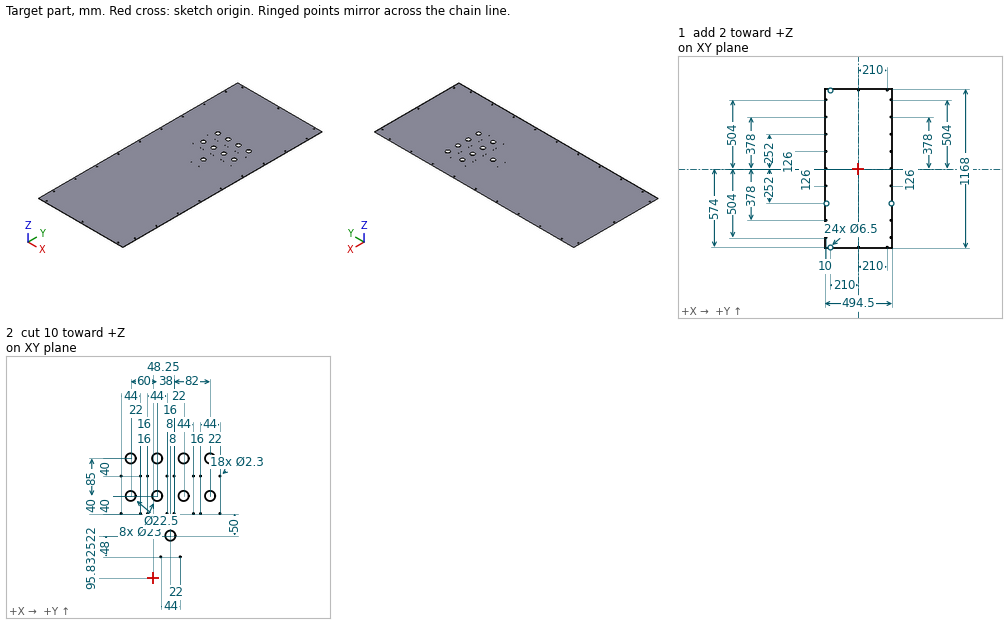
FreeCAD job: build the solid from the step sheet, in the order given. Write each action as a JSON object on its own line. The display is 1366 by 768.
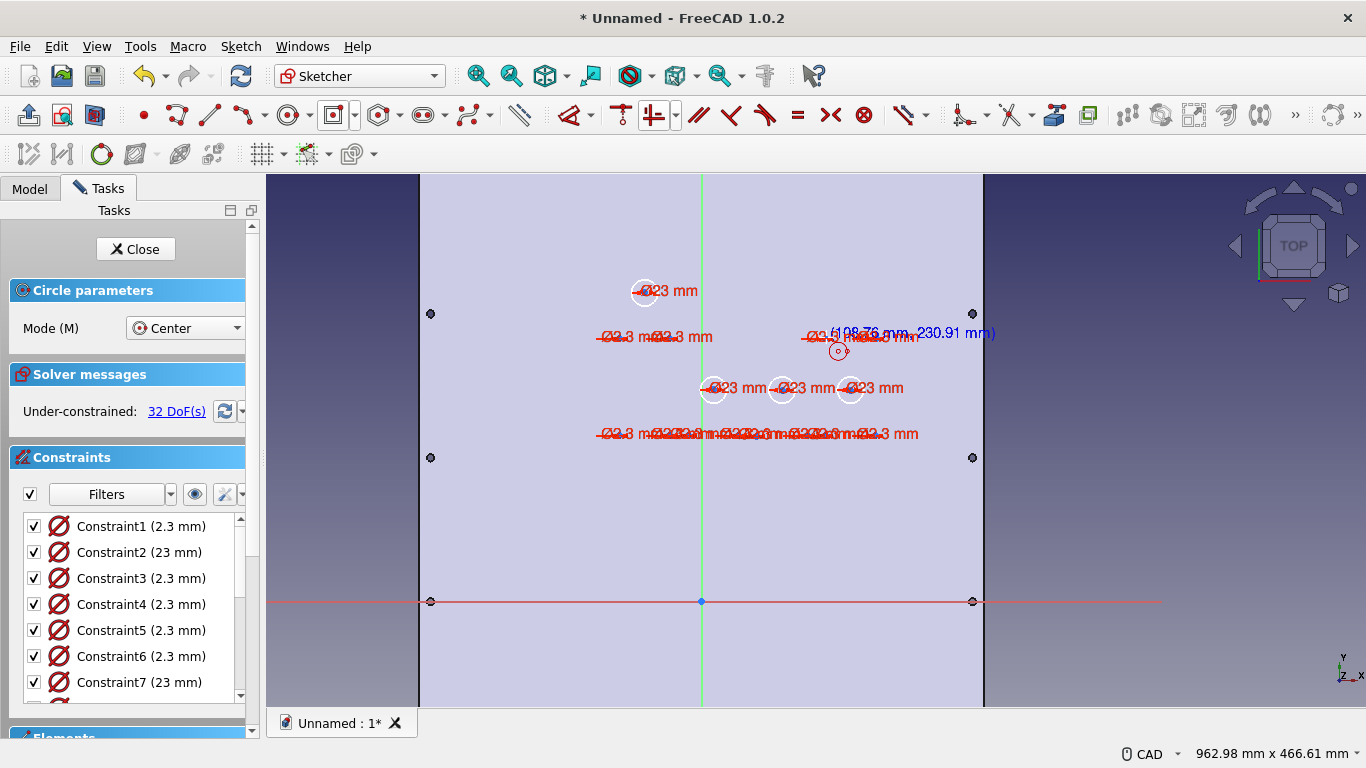
{"action": "scroll", "coordinate": [782, 292], "scroll_direction": "up", "scroll_amount": 3}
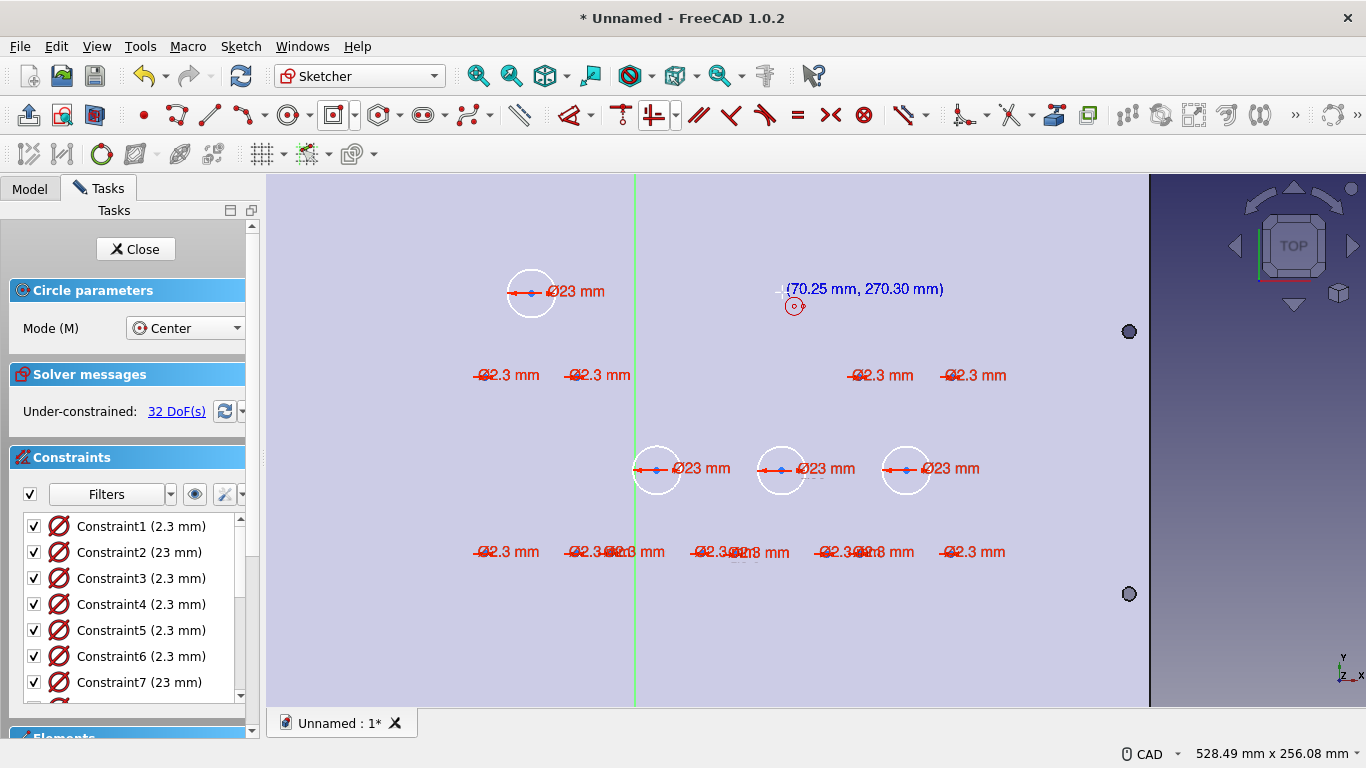
{"action": "left_click", "coordinate": [782, 293]}
{"action": "mouse_move", "coordinate": [799, 276]}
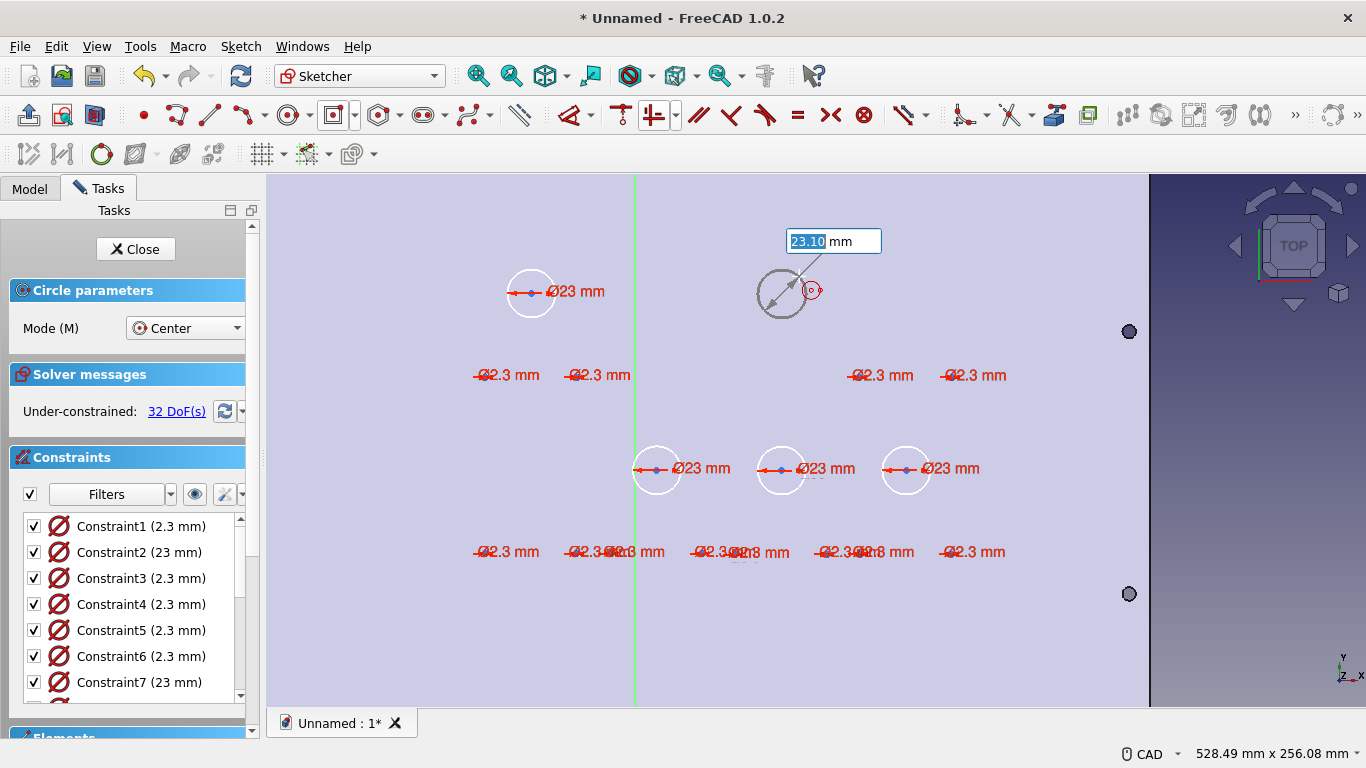
{"action": "type", "text": "23"}
{"action": "key", "text": "Return"}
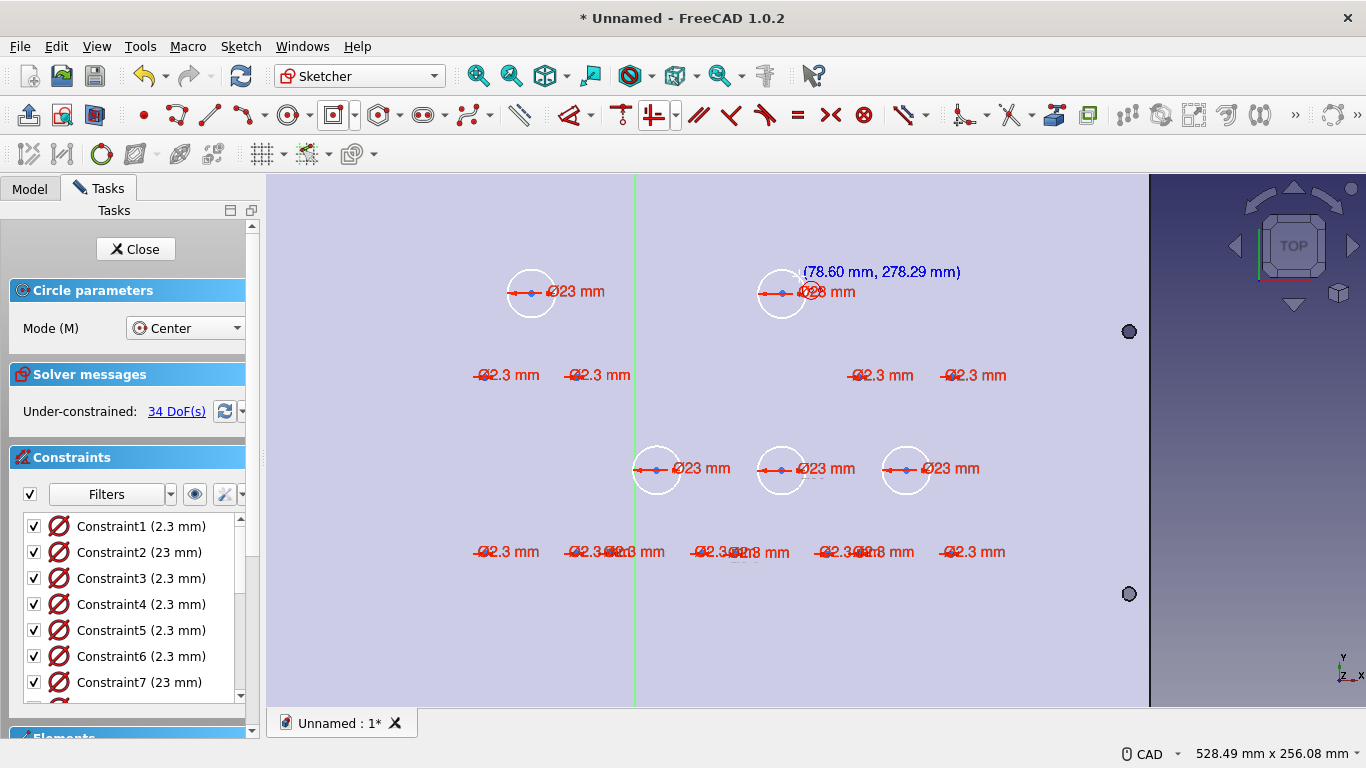
{"action": "scroll", "coordinate": [827, 376], "scroll_direction": "up", "scroll_amount": 12}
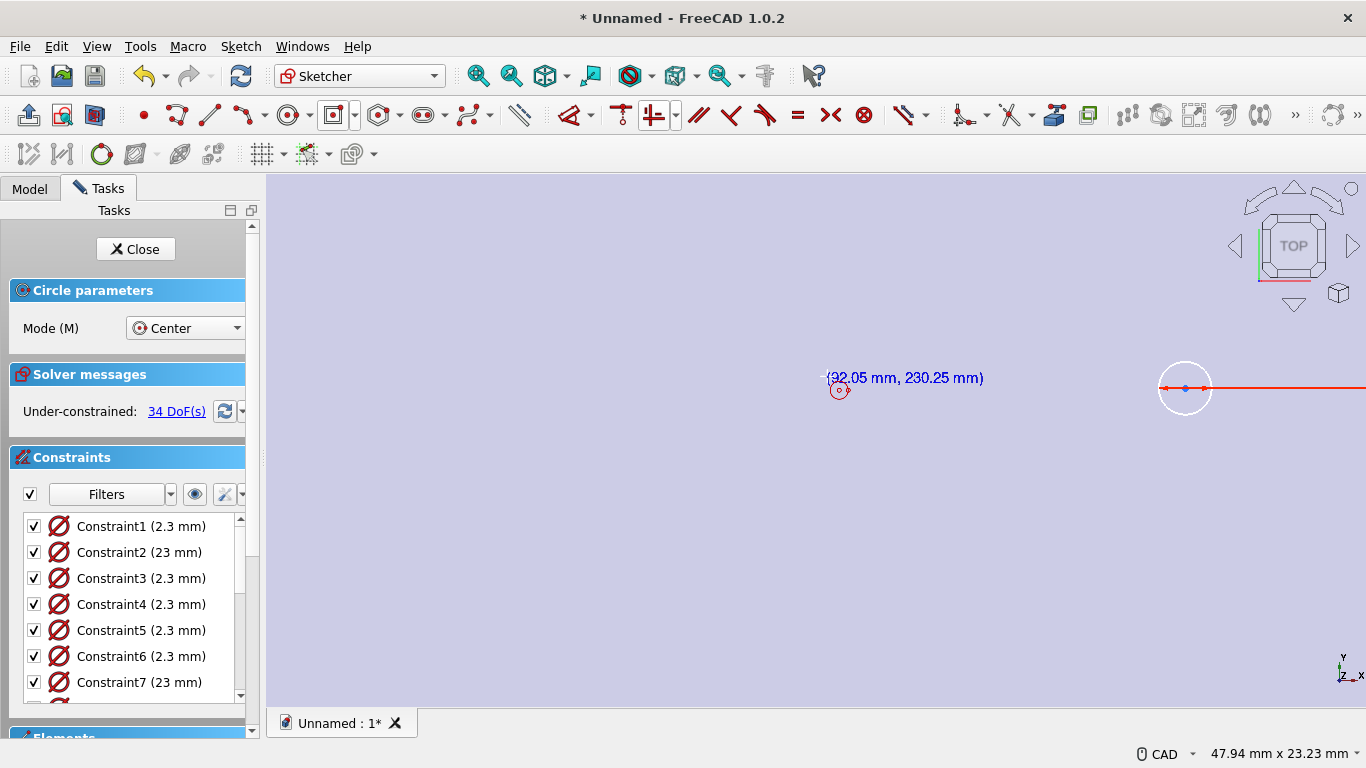
{"action": "scroll", "coordinate": [806, 336], "scroll_direction": "down", "scroll_amount": 15}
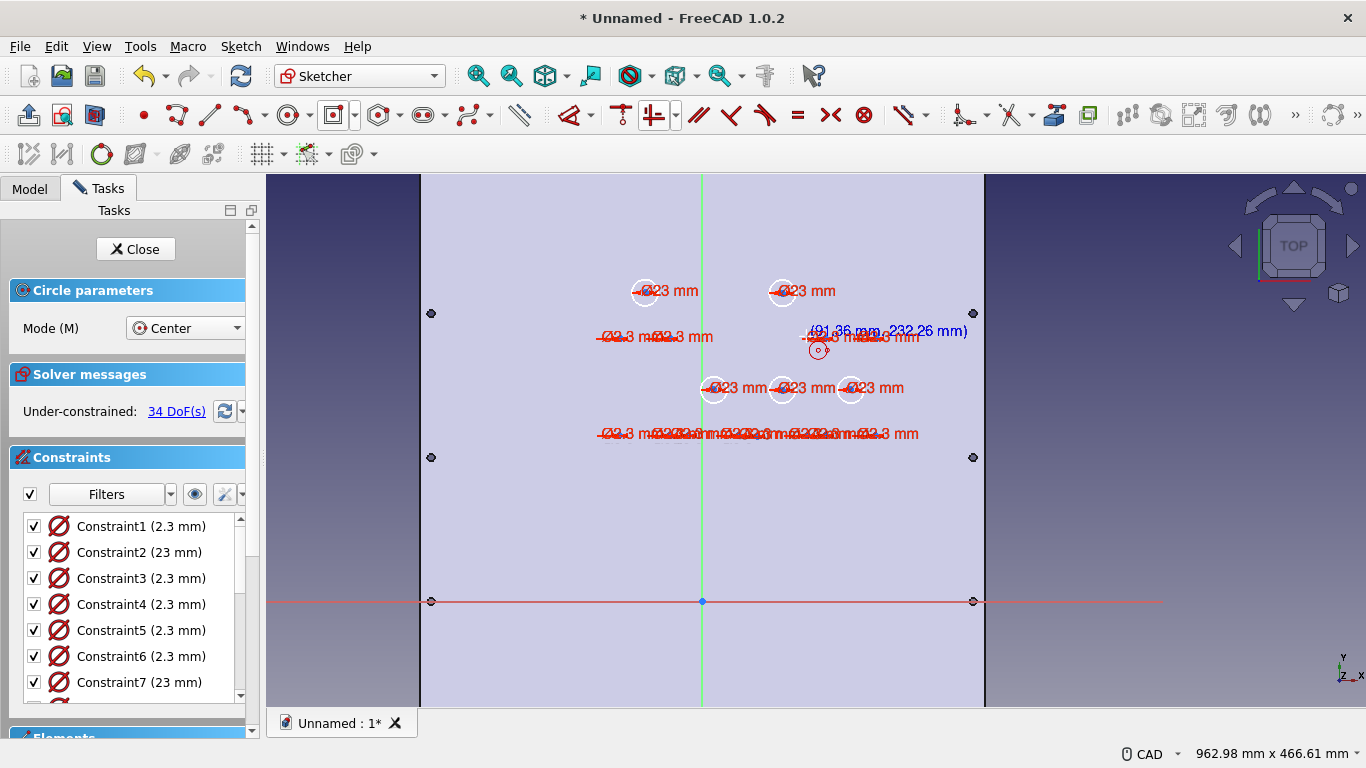
{"action": "left_click", "coordinate": [807, 338]}
{"action": "mouse_move", "coordinate": [808, 337]}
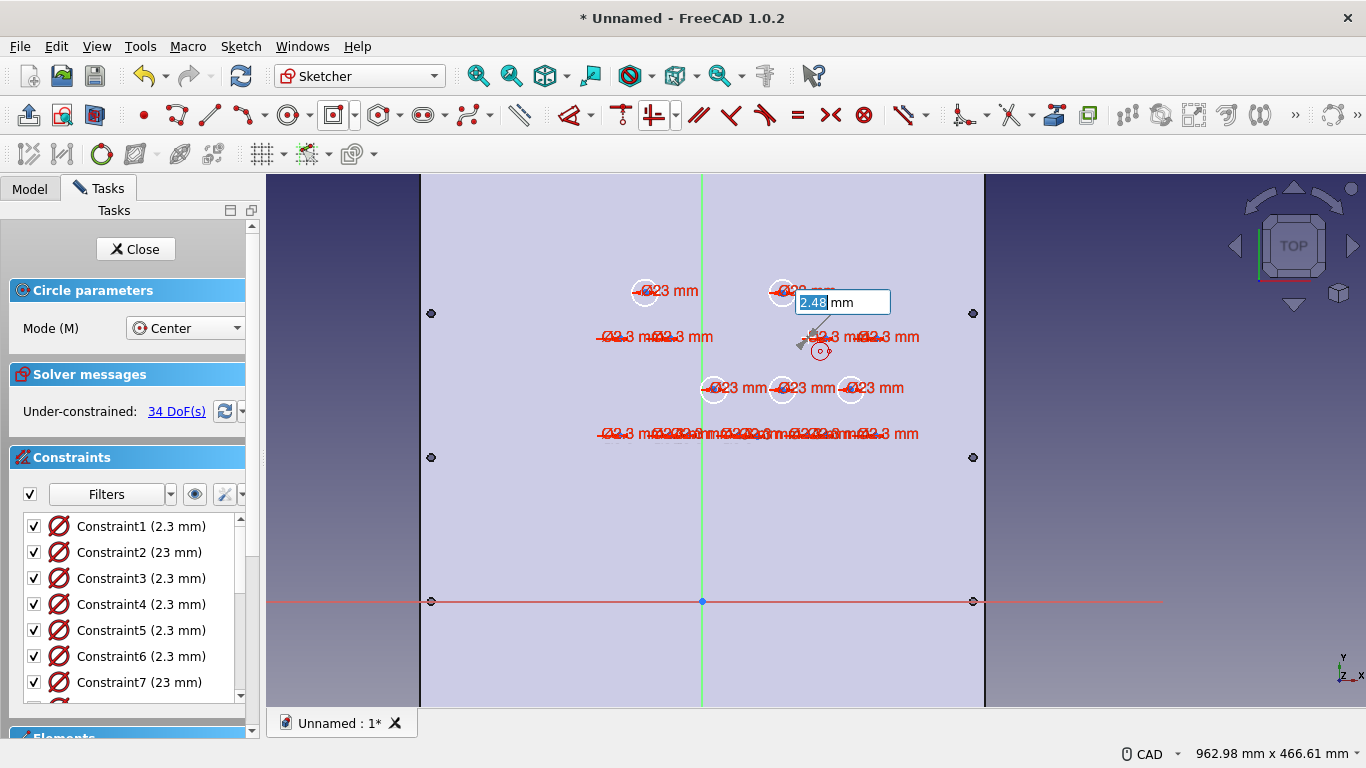
{"action": "type", "text": "2.3"}
{"action": "key", "text": "Return"}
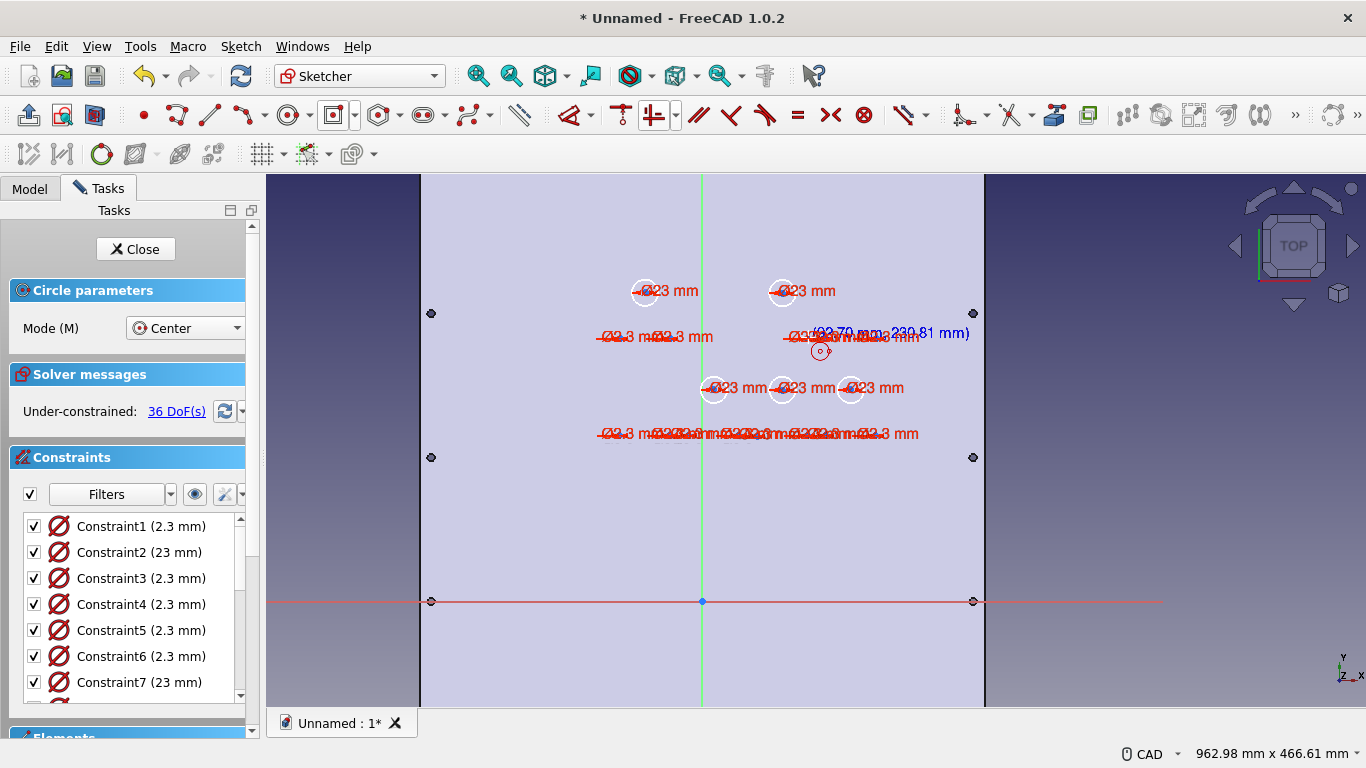
{"action": "scroll", "coordinate": [757, 338], "scroll_direction": "up", "scroll_amount": 15}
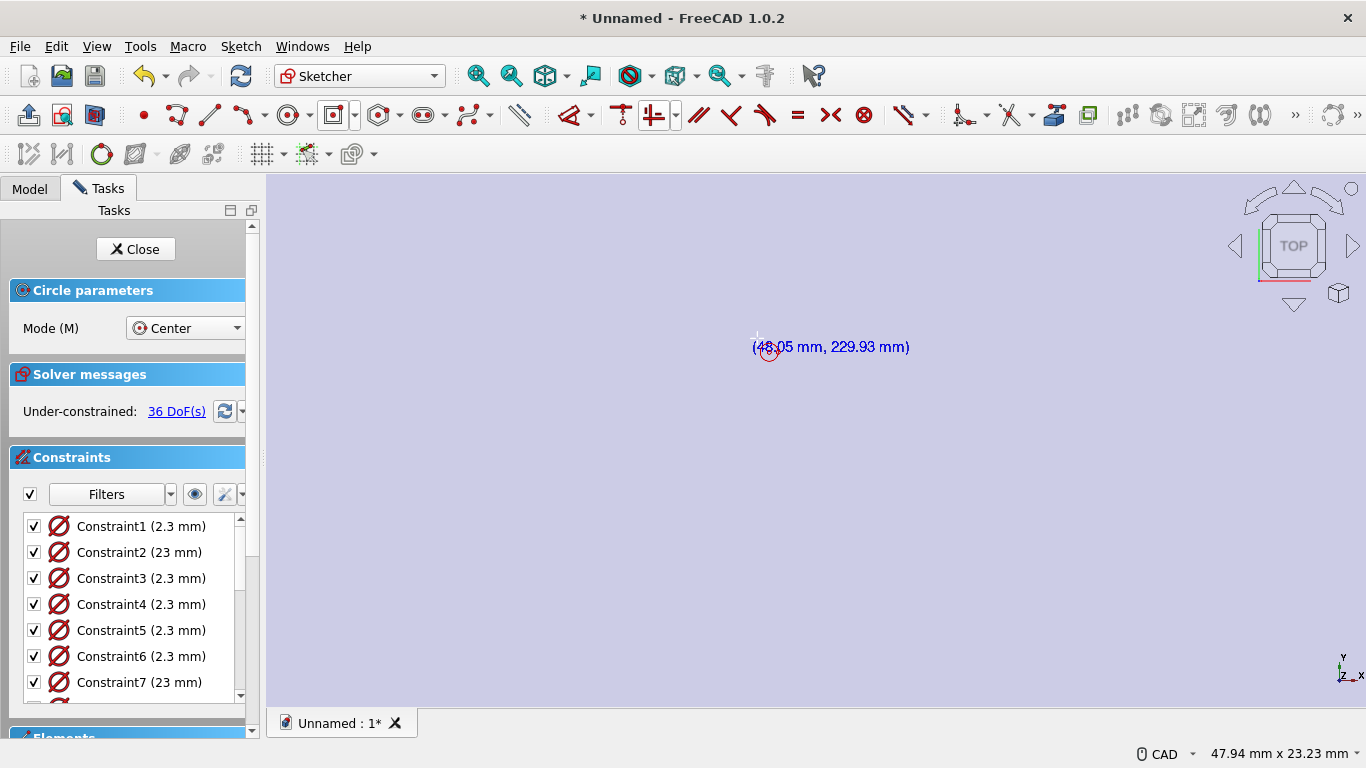
{"action": "scroll", "coordinate": [757, 338], "scroll_direction": "down", "scroll_amount": 15}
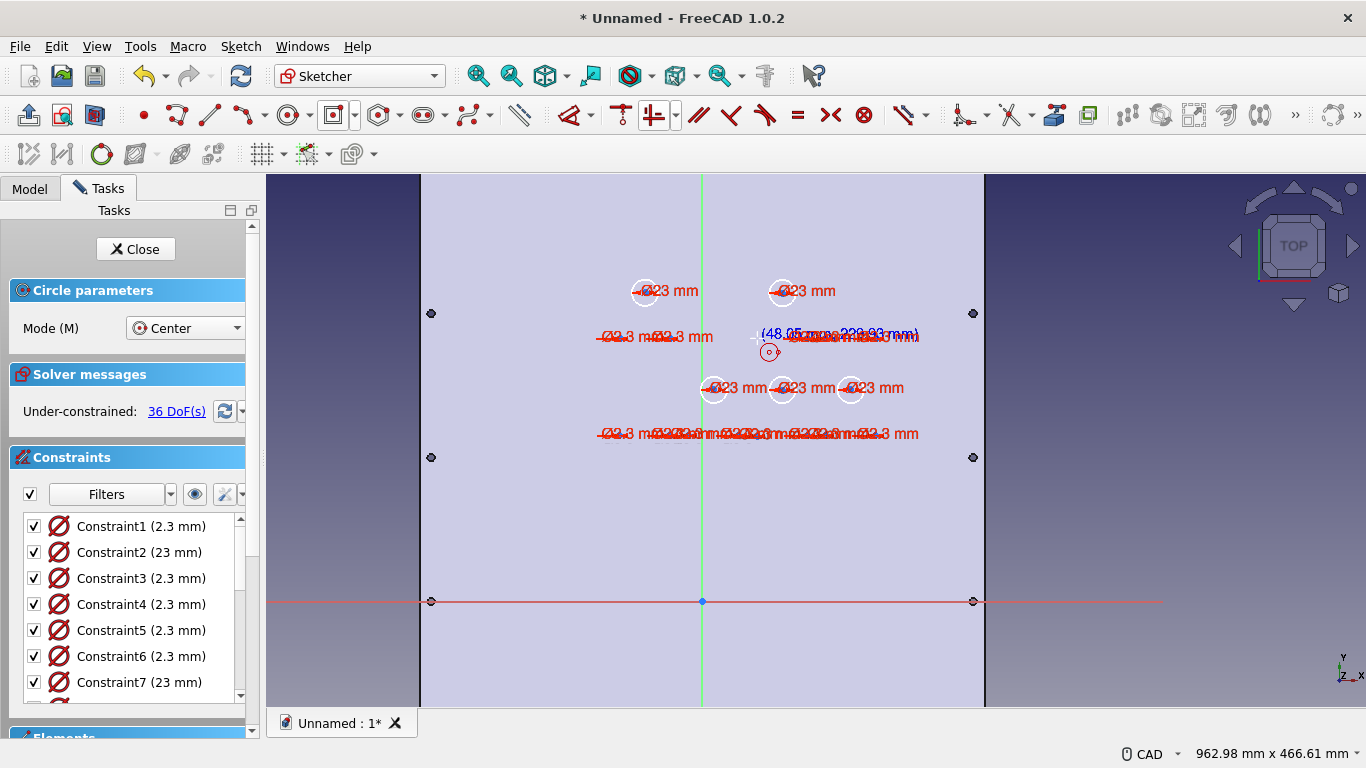
{"action": "left_click", "coordinate": [757, 338]}
{"action": "mouse_move", "coordinate": [758, 337]}